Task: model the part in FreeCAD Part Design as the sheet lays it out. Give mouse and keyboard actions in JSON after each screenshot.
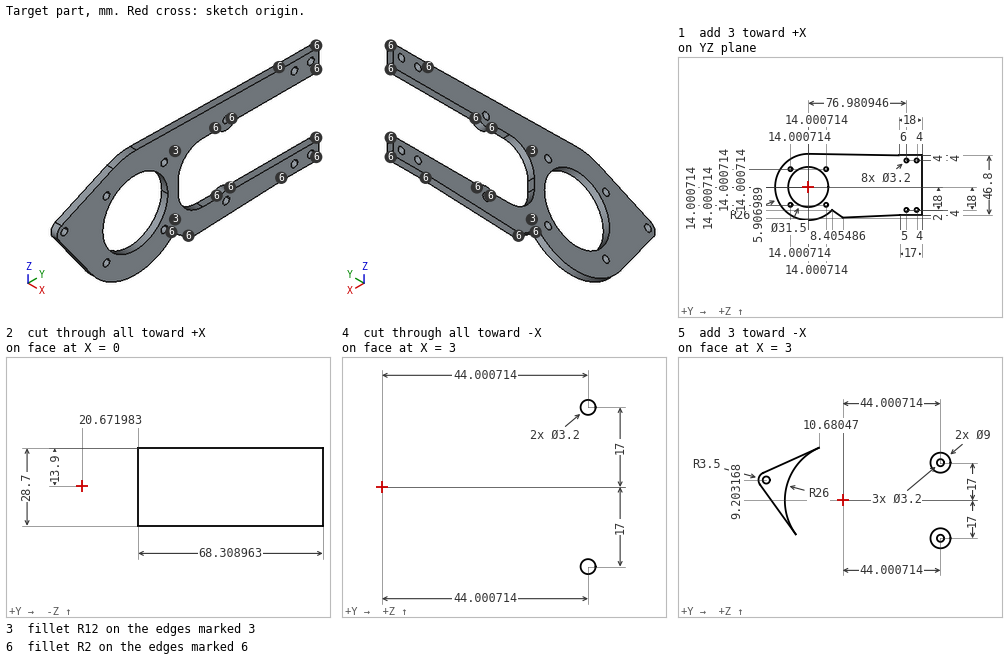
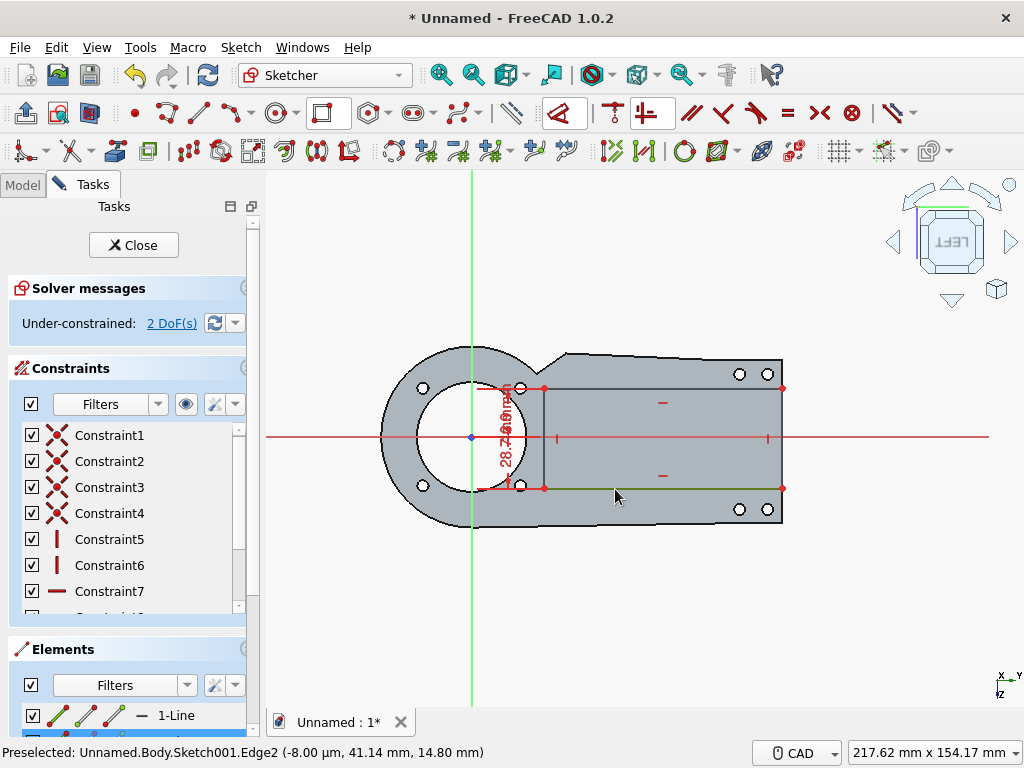
{"action": "left_click", "coordinate": [582, 114]}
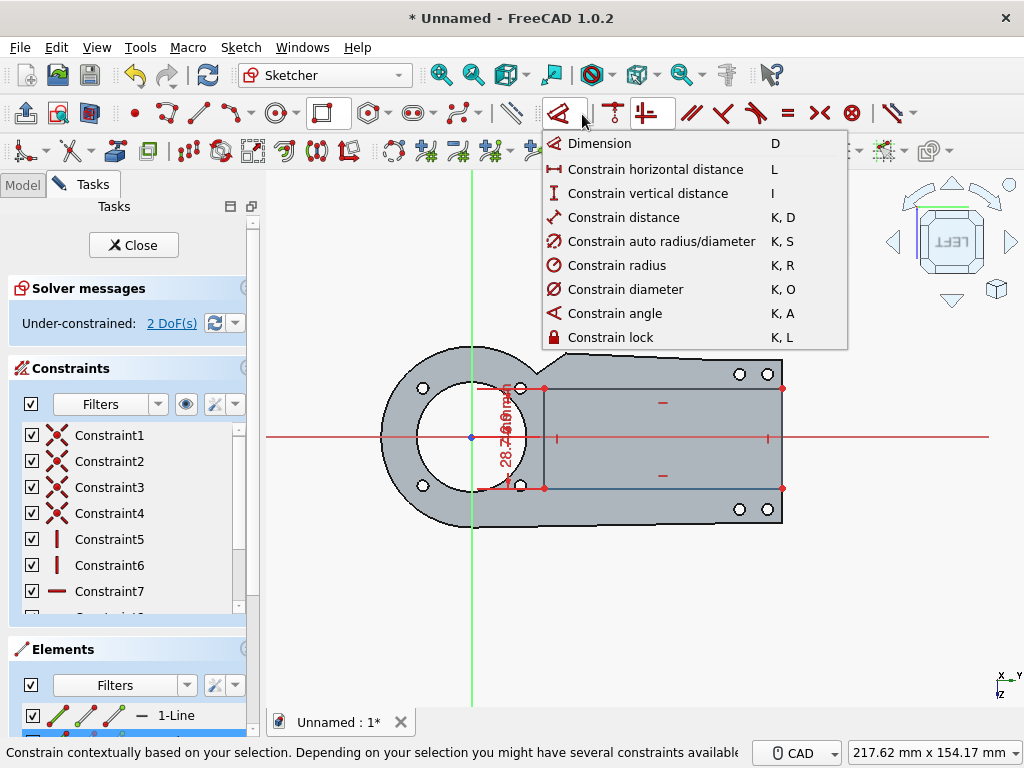
{"action": "left_click", "coordinate": [695, 169]}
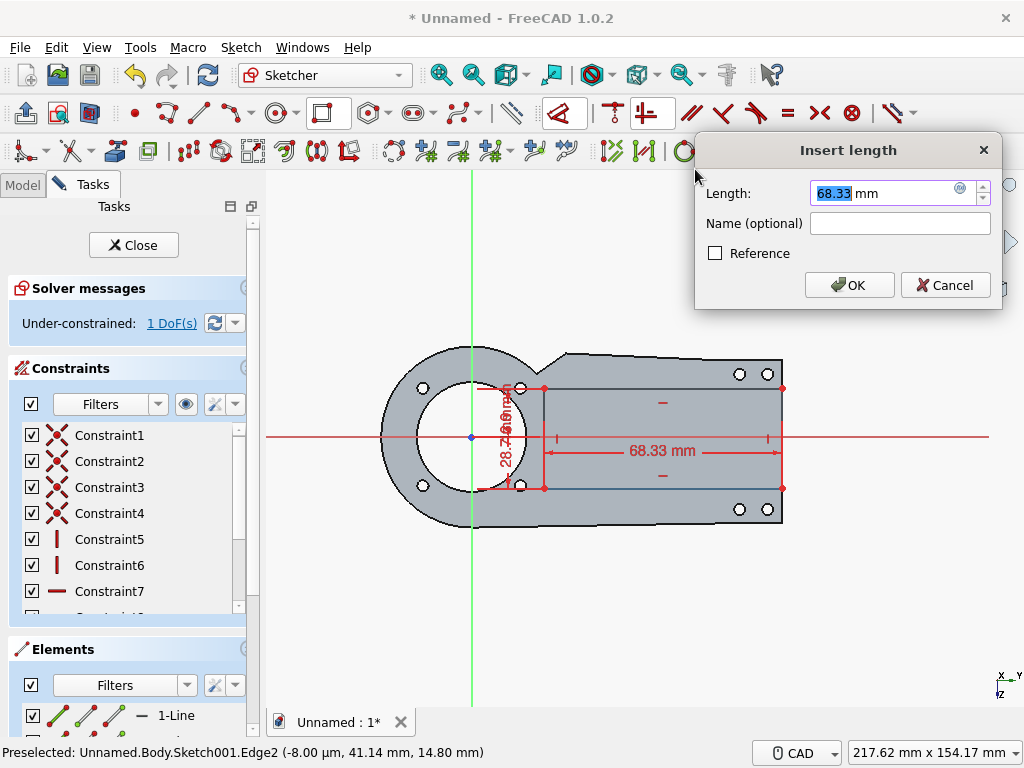
{"action": "type", "text": "68.308963"}
{"action": "key", "text": "Return"}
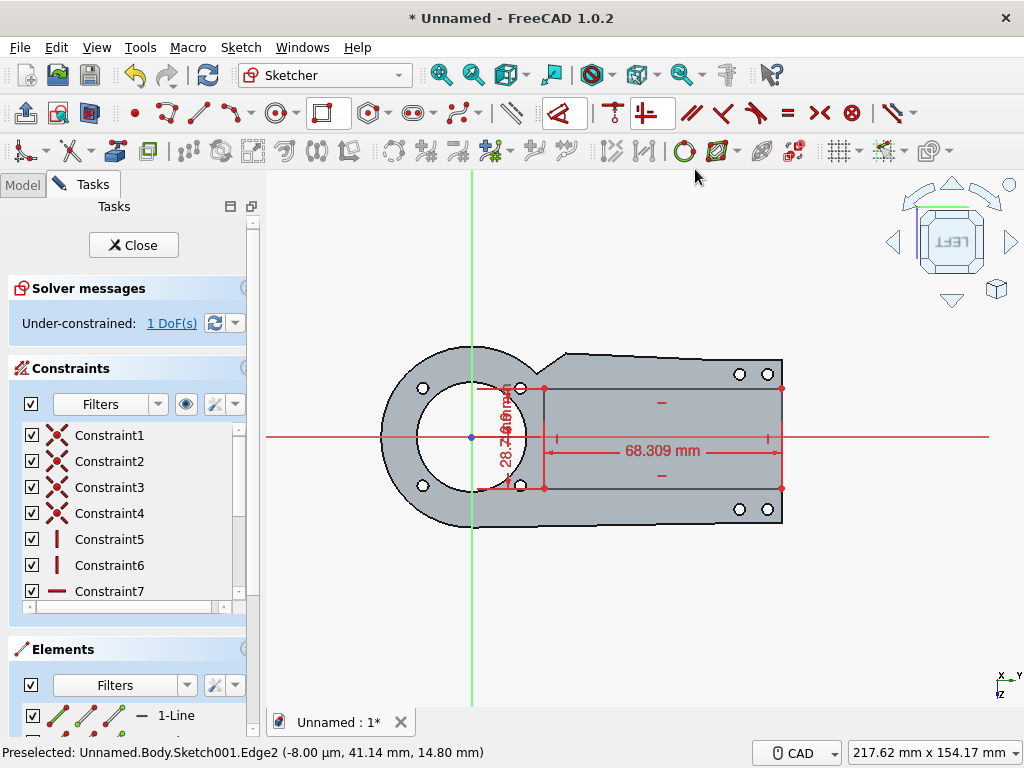
{"action": "left_click", "coordinate": [544, 389]}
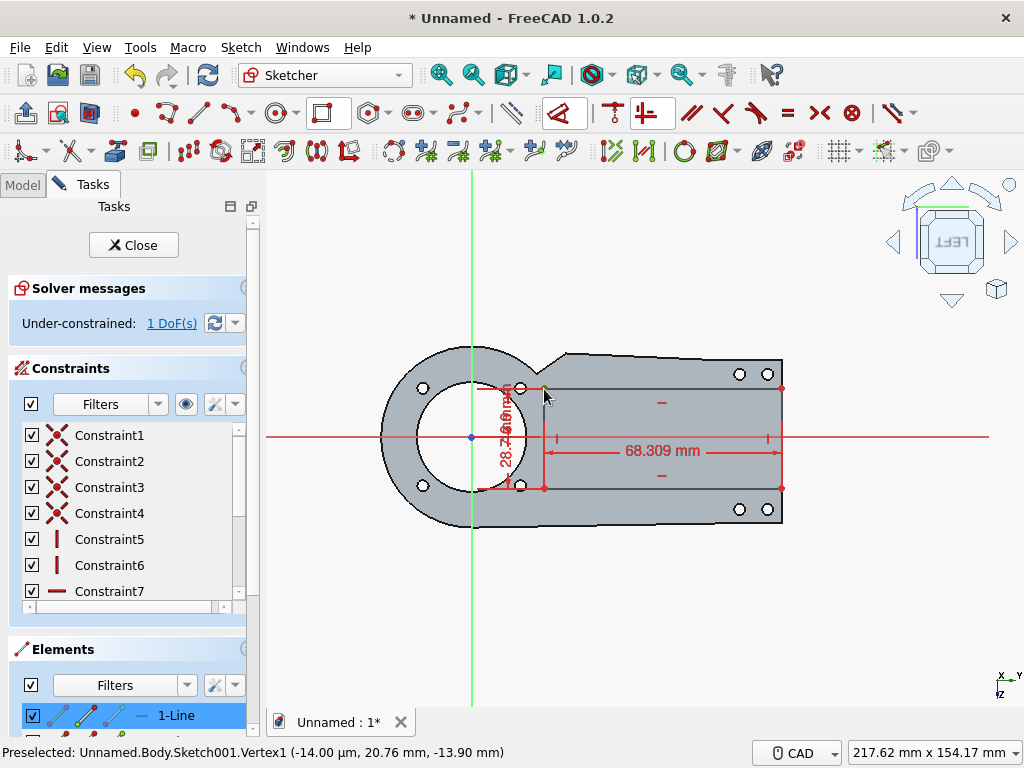
{"action": "left_click", "coordinate": [582, 114]}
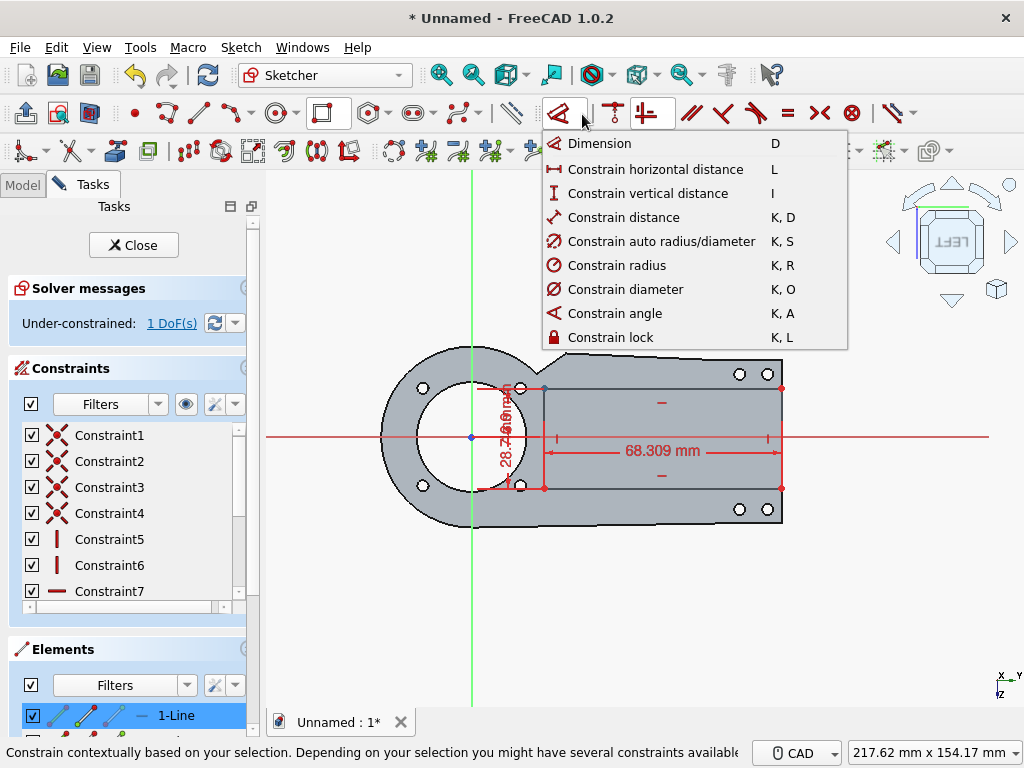
{"action": "left_click", "coordinate": [695, 169]}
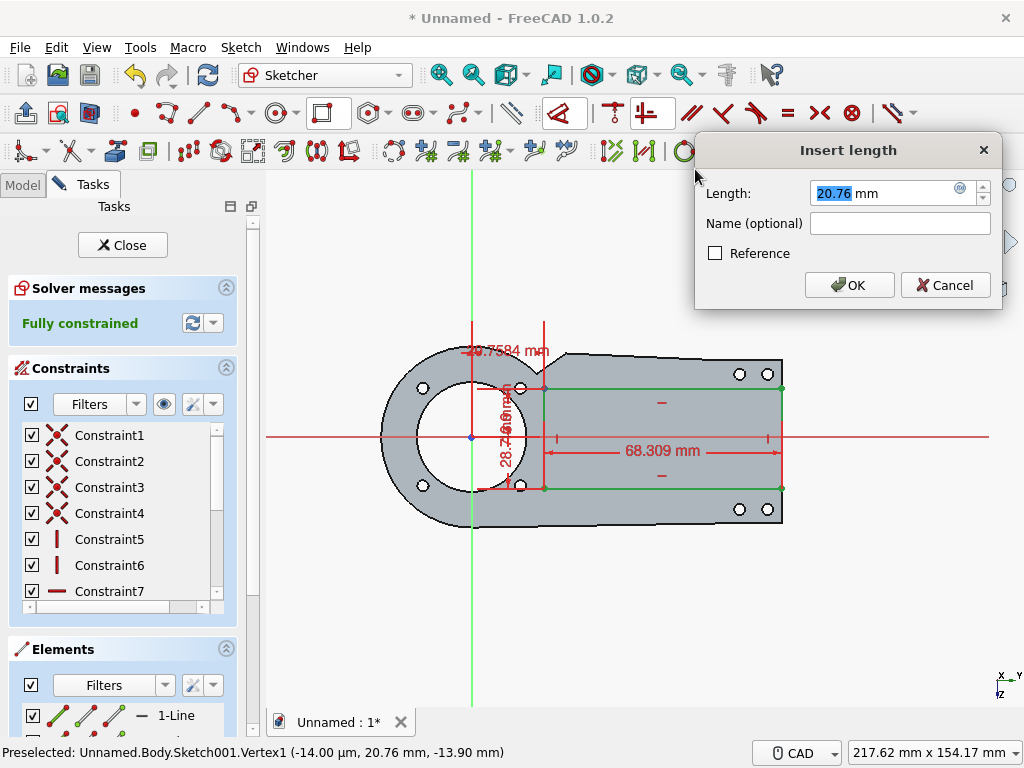
{"action": "type", "text": "20.671983"}
{"action": "key", "text": "Return"}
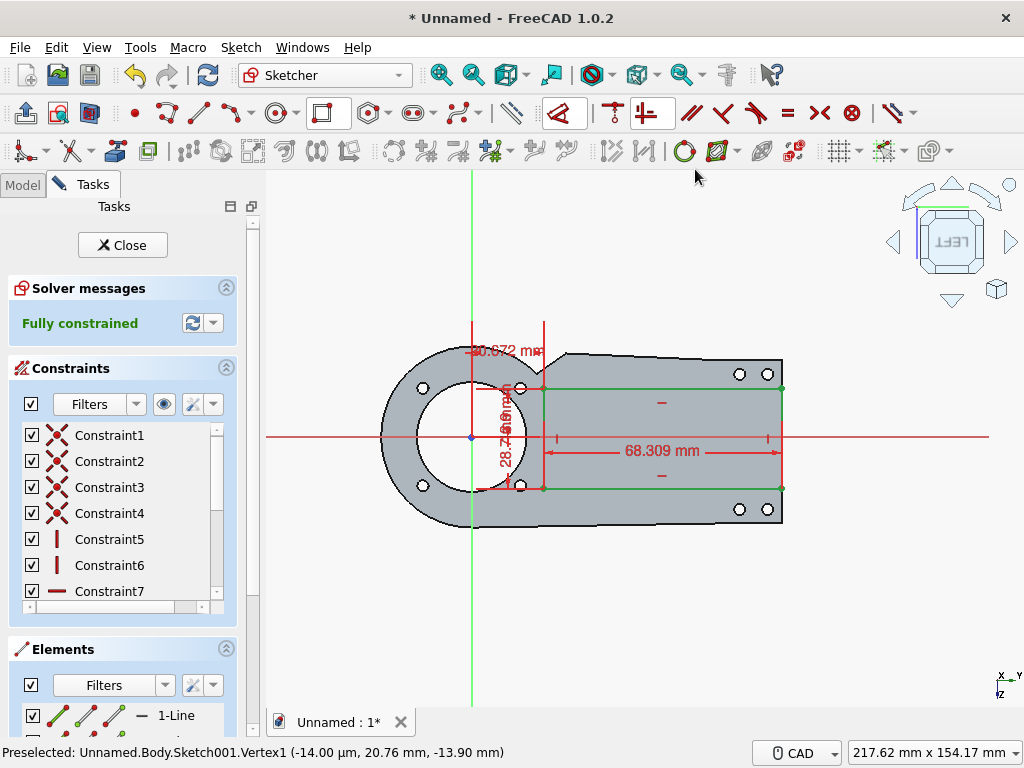
{"action": "left_click", "coordinate": [123, 245]}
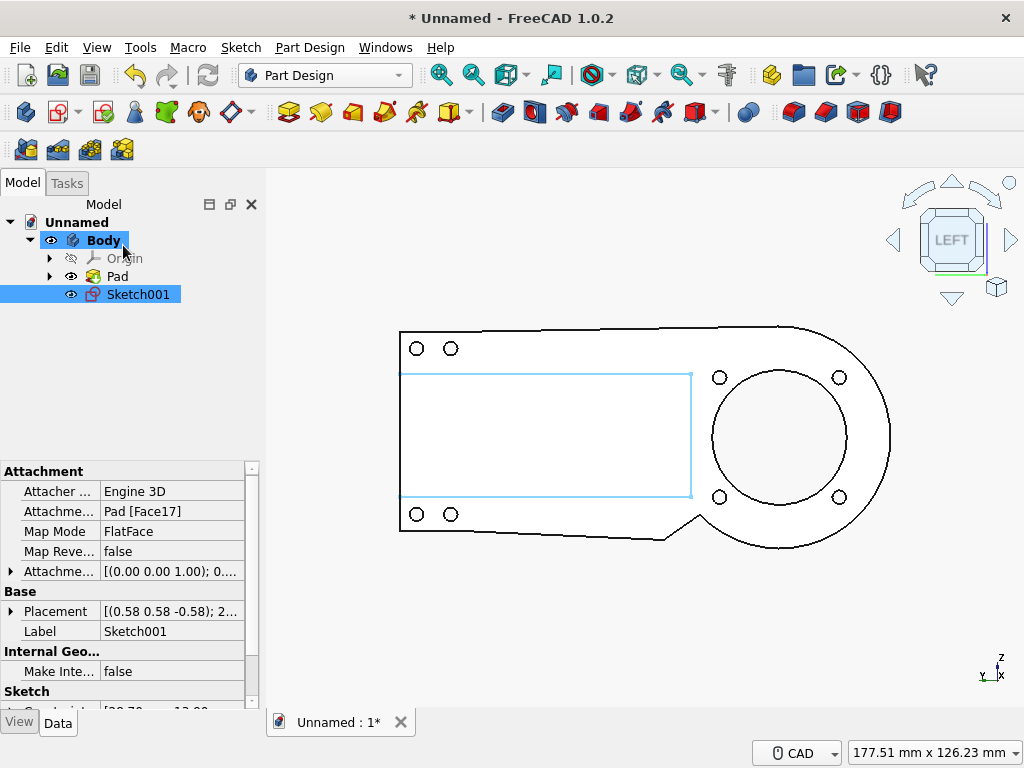
{"action": "left_click", "coordinate": [504, 112]}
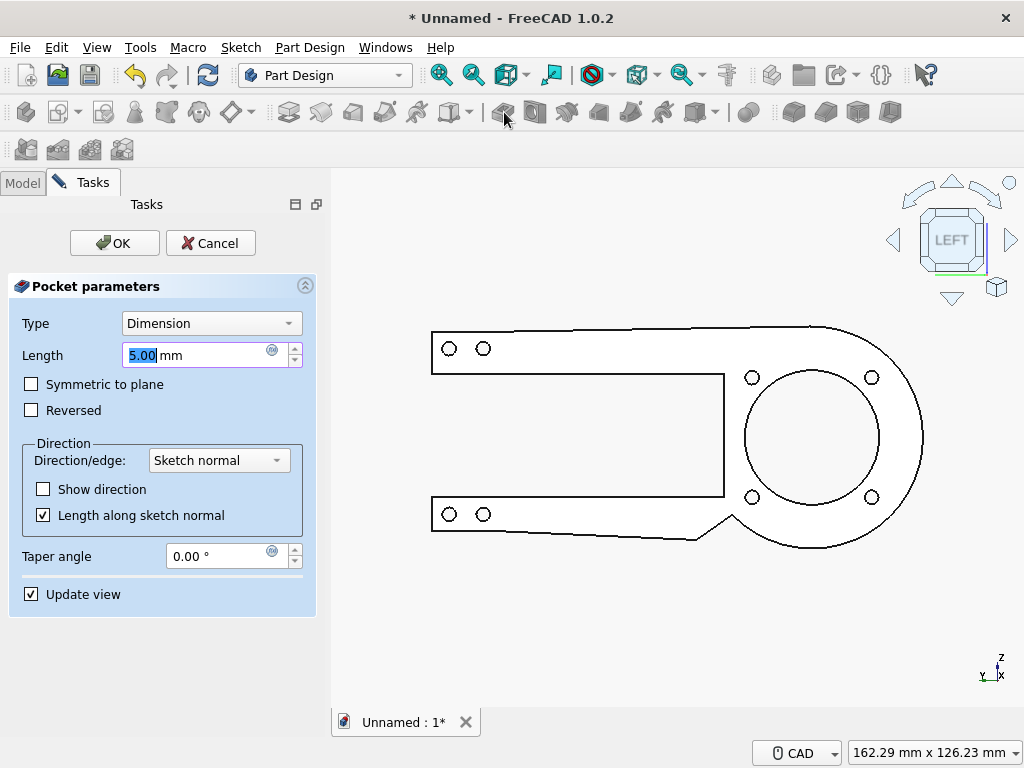
{"action": "left_click", "coordinate": [212, 324]}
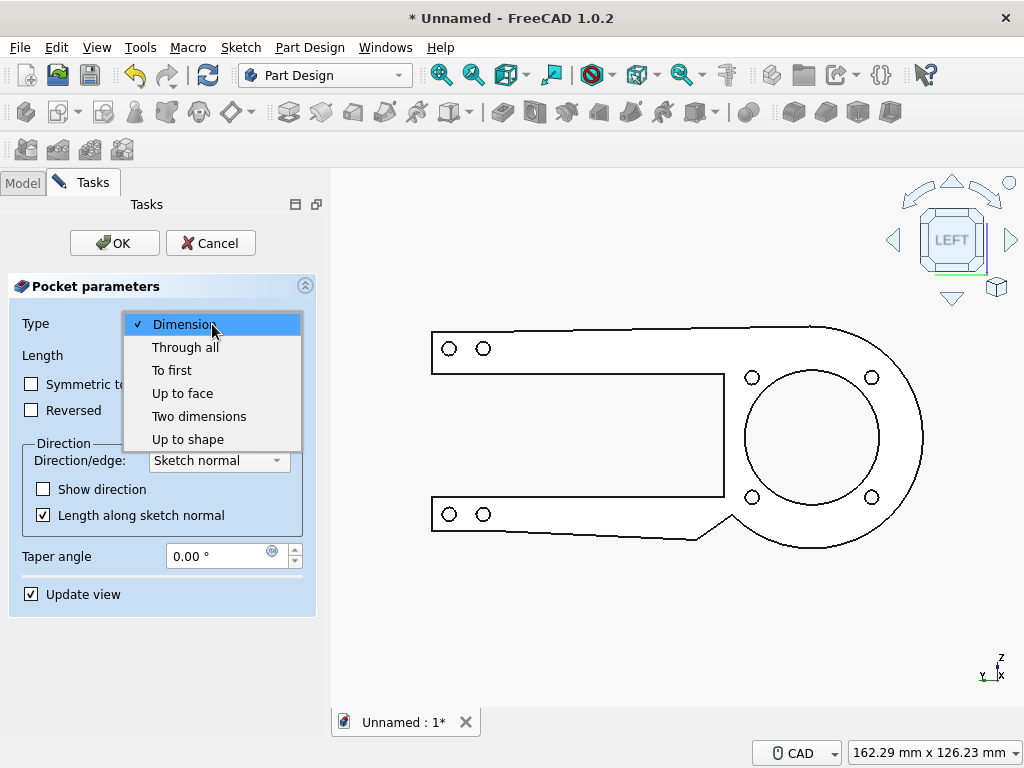
{"action": "left_click", "coordinate": [212, 348]}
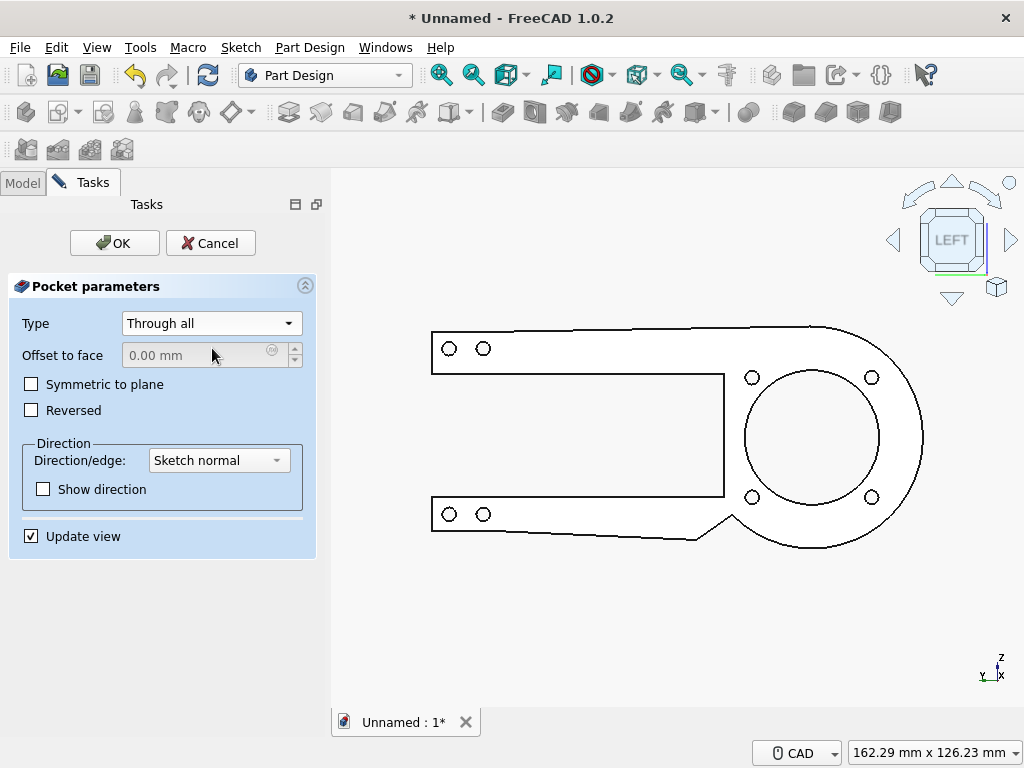
{"action": "left_click", "coordinate": [115, 243]}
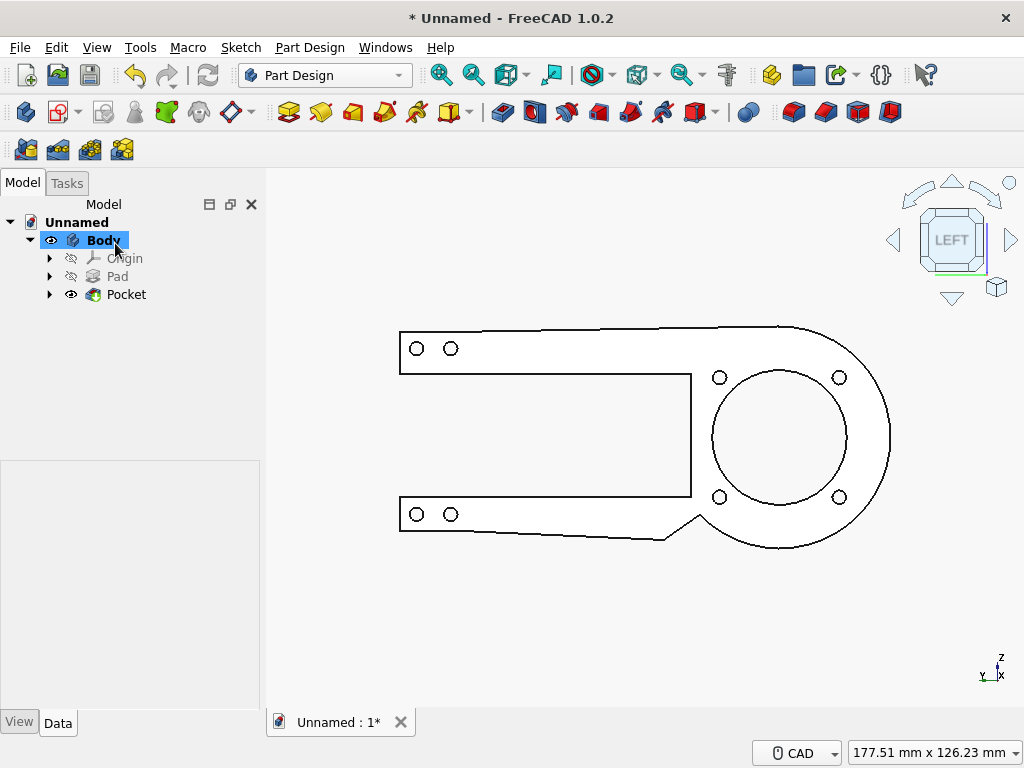
{"action": "scroll", "coordinate": [691, 496], "scroll_direction": "up", "scroll_amount": 6}